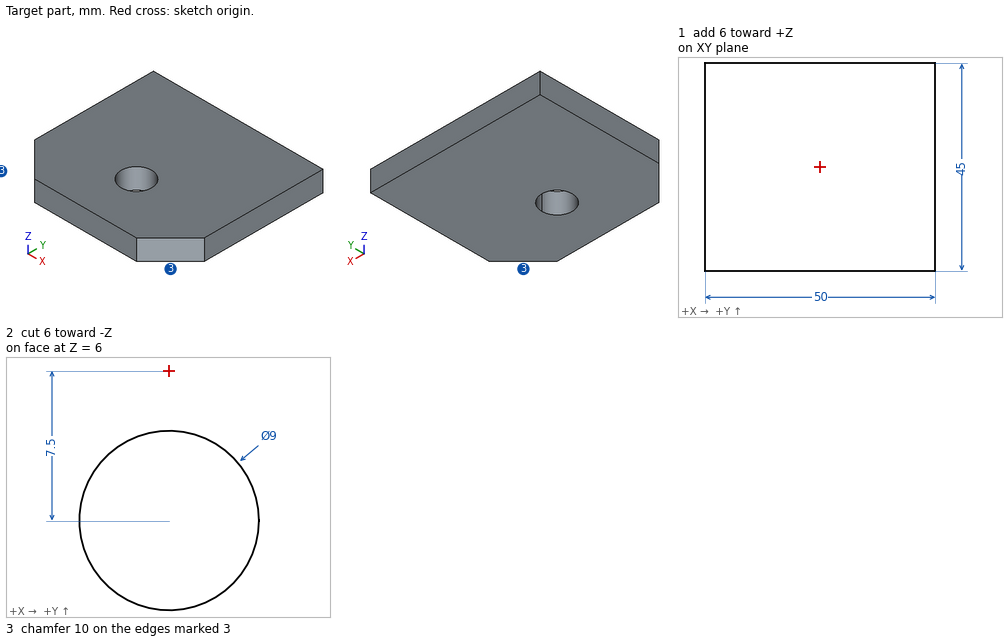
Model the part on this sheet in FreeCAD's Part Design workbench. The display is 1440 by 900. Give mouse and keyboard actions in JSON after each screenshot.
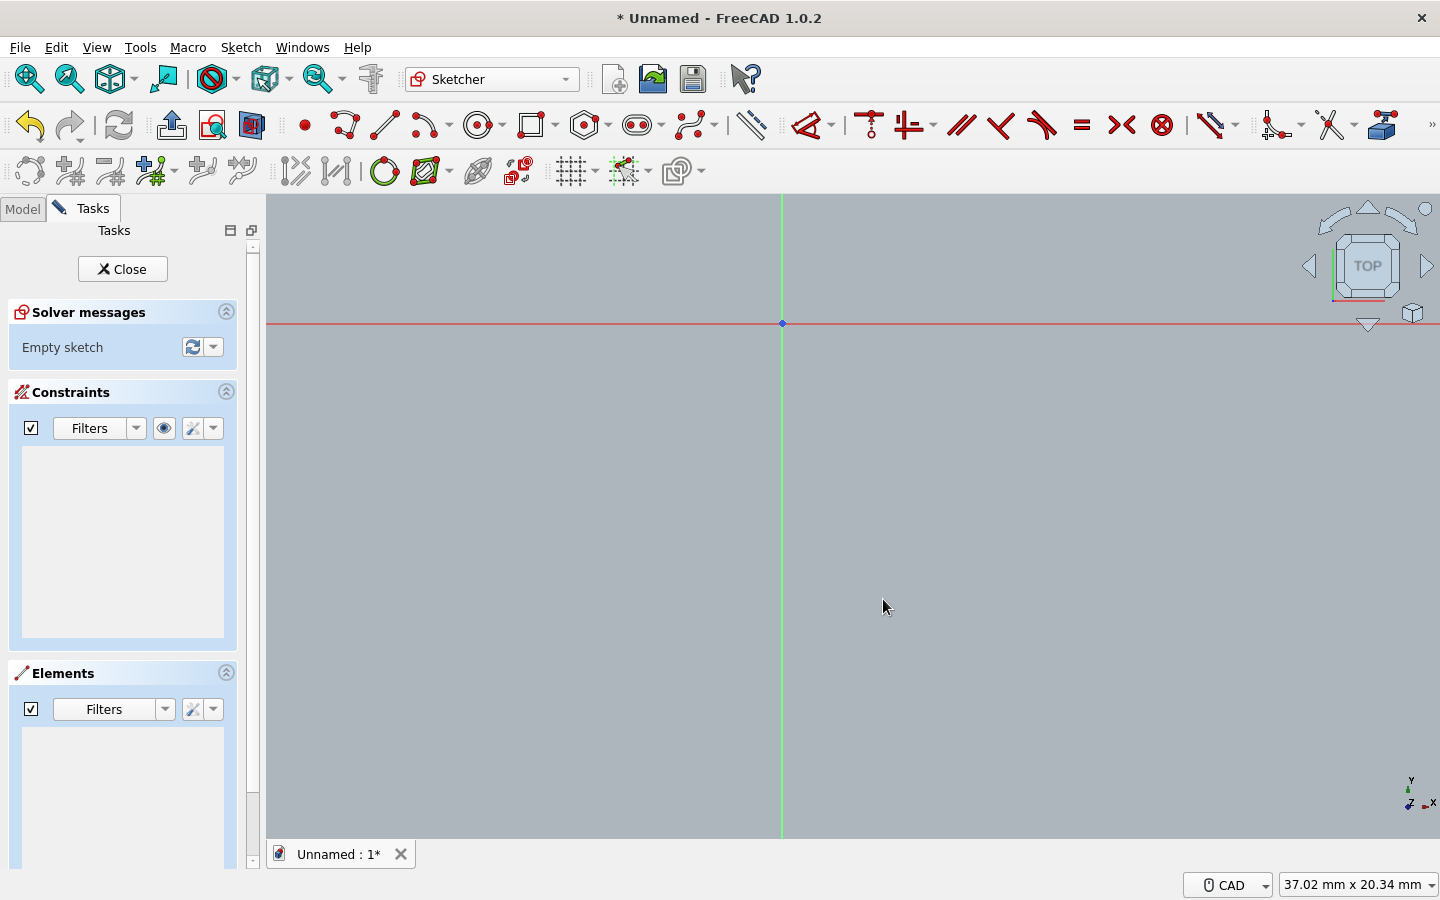
{"action": "key", "text": "g c"}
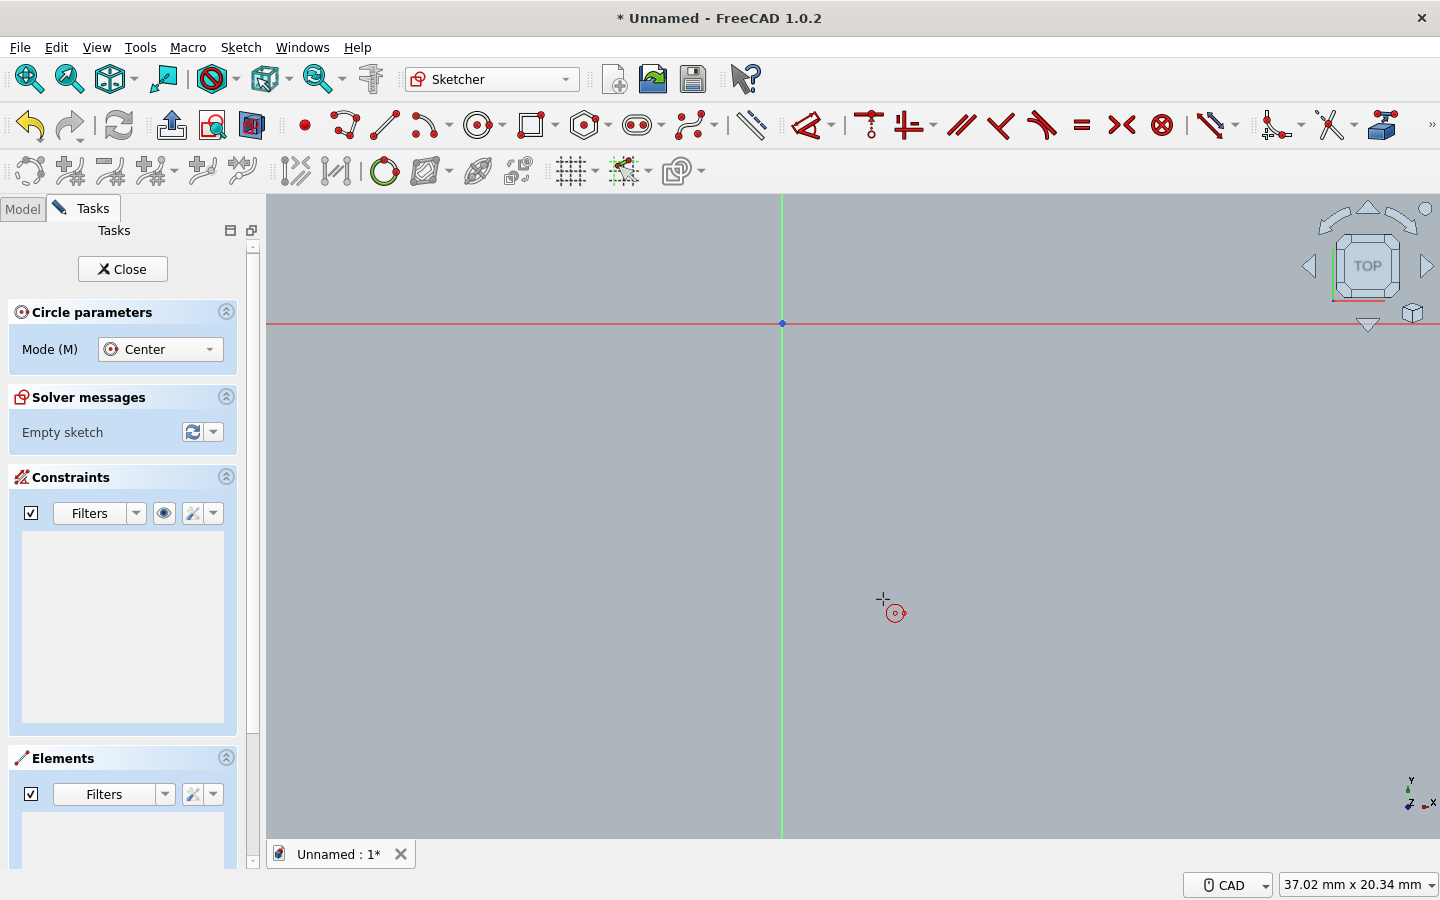
{"action": "left_click", "coordinate": [782, 561]}
{"action": "mouse_move", "coordinate": [883, 461]}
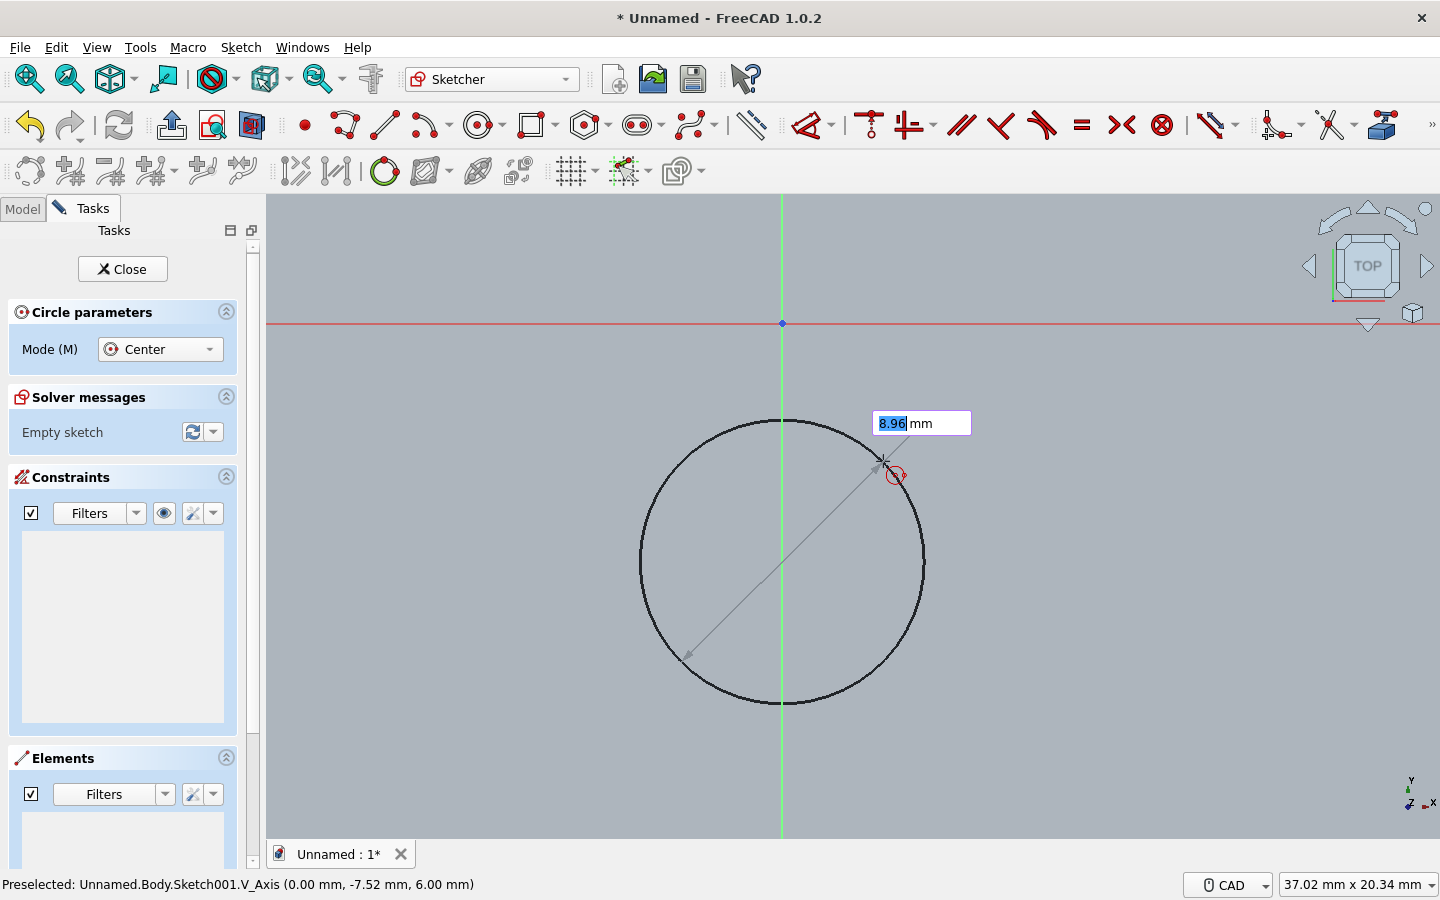
{"action": "type", "text": "9"}
{"action": "key", "text": "Return"}
{"action": "key", "text": "Escape"}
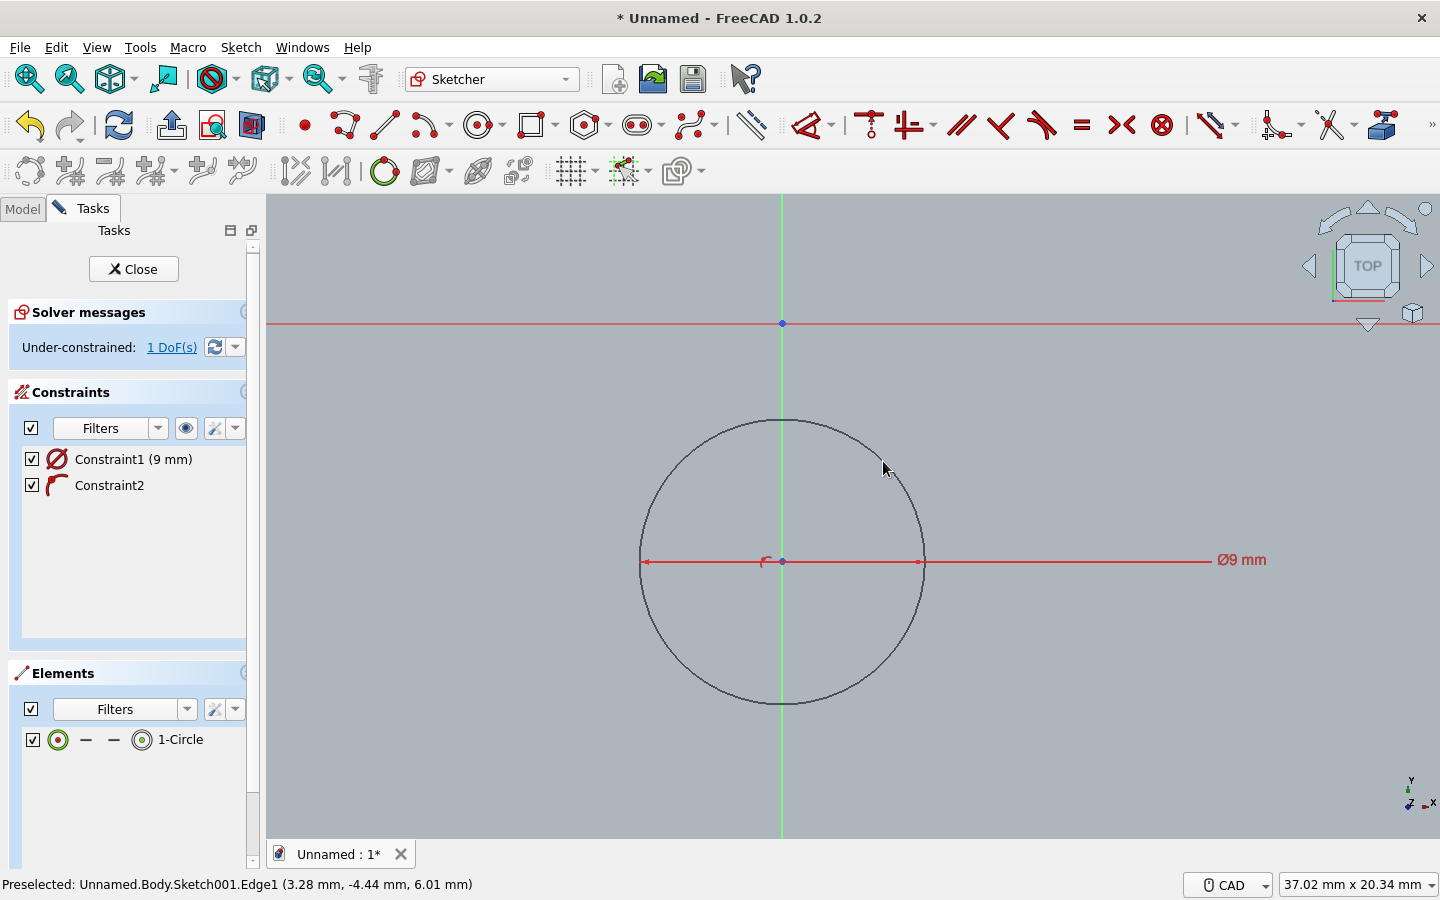
{"action": "left_click", "coordinate": [806, 126]}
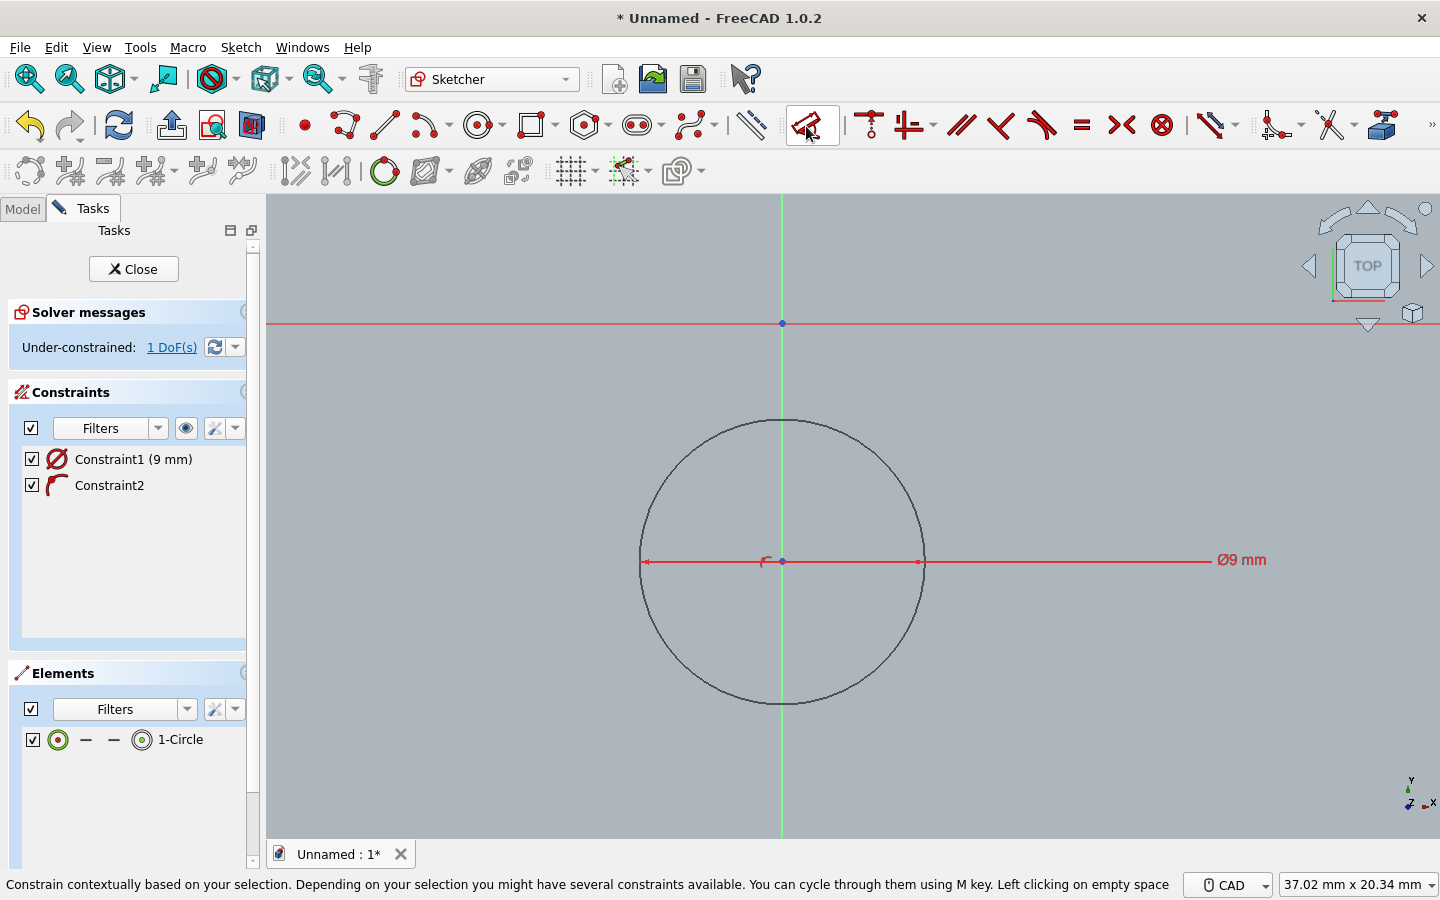
{"action": "left_click", "coordinate": [782, 562]}
{"action": "left_click", "coordinate": [816, 443]}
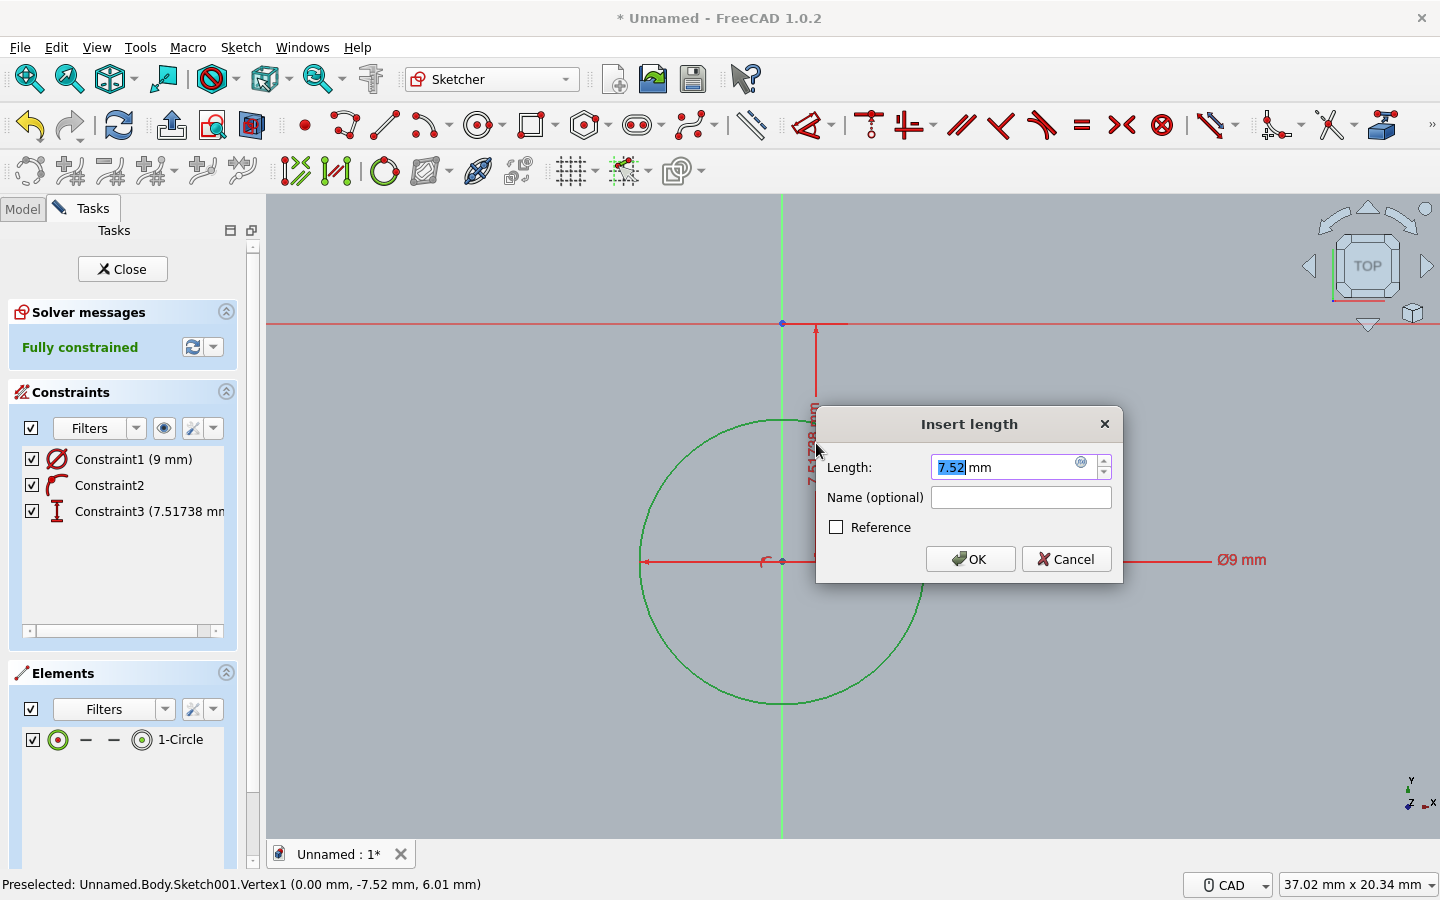
{"action": "type", "text": "7.5"}
{"action": "key", "text": "Return"}
{"action": "key", "text": "Escape"}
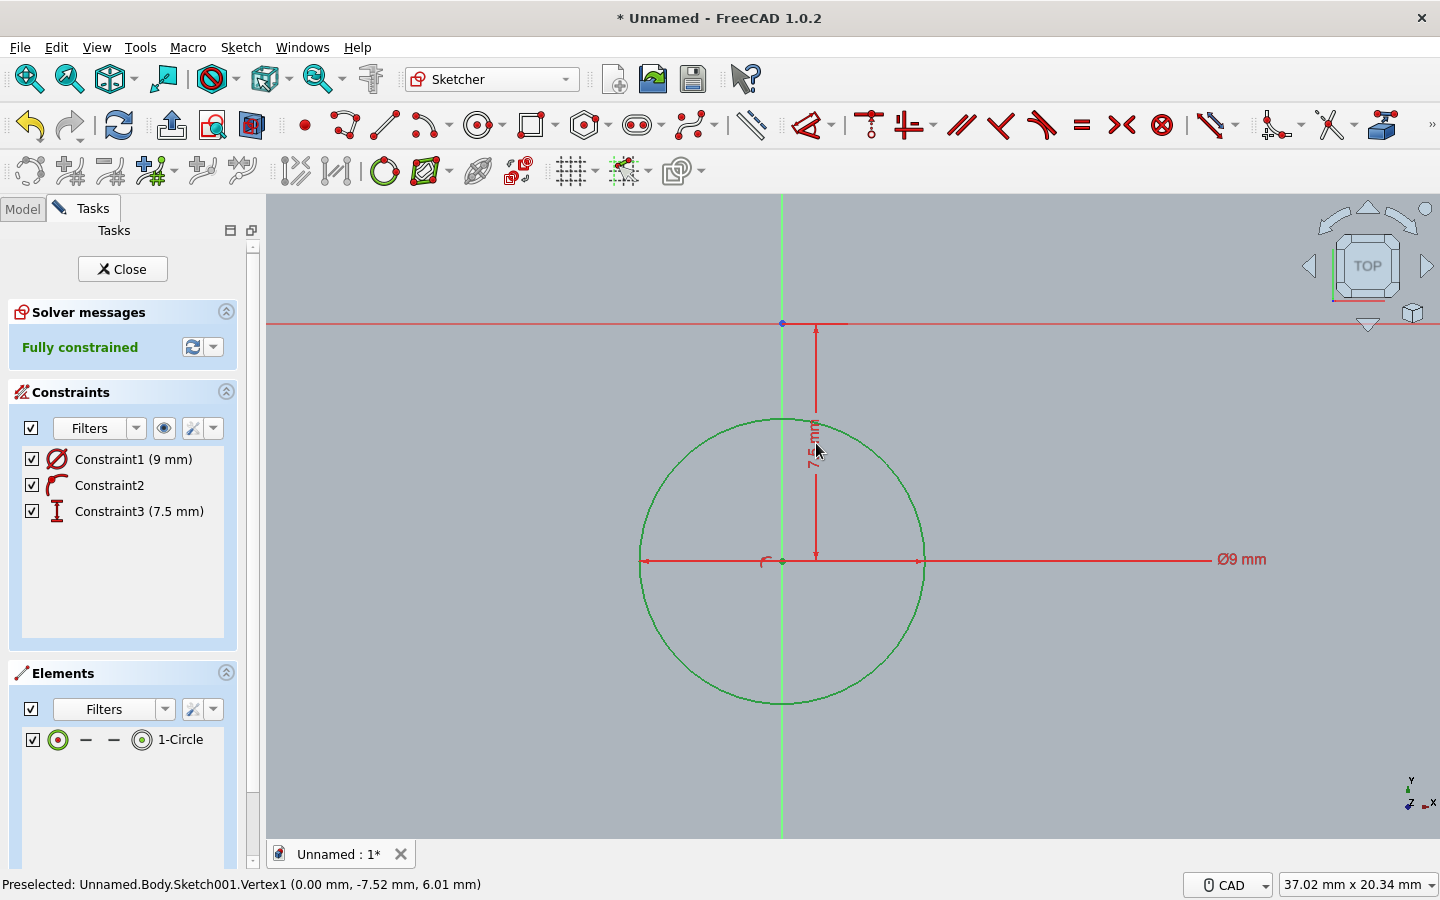
{"action": "left_click", "coordinate": [123, 269]}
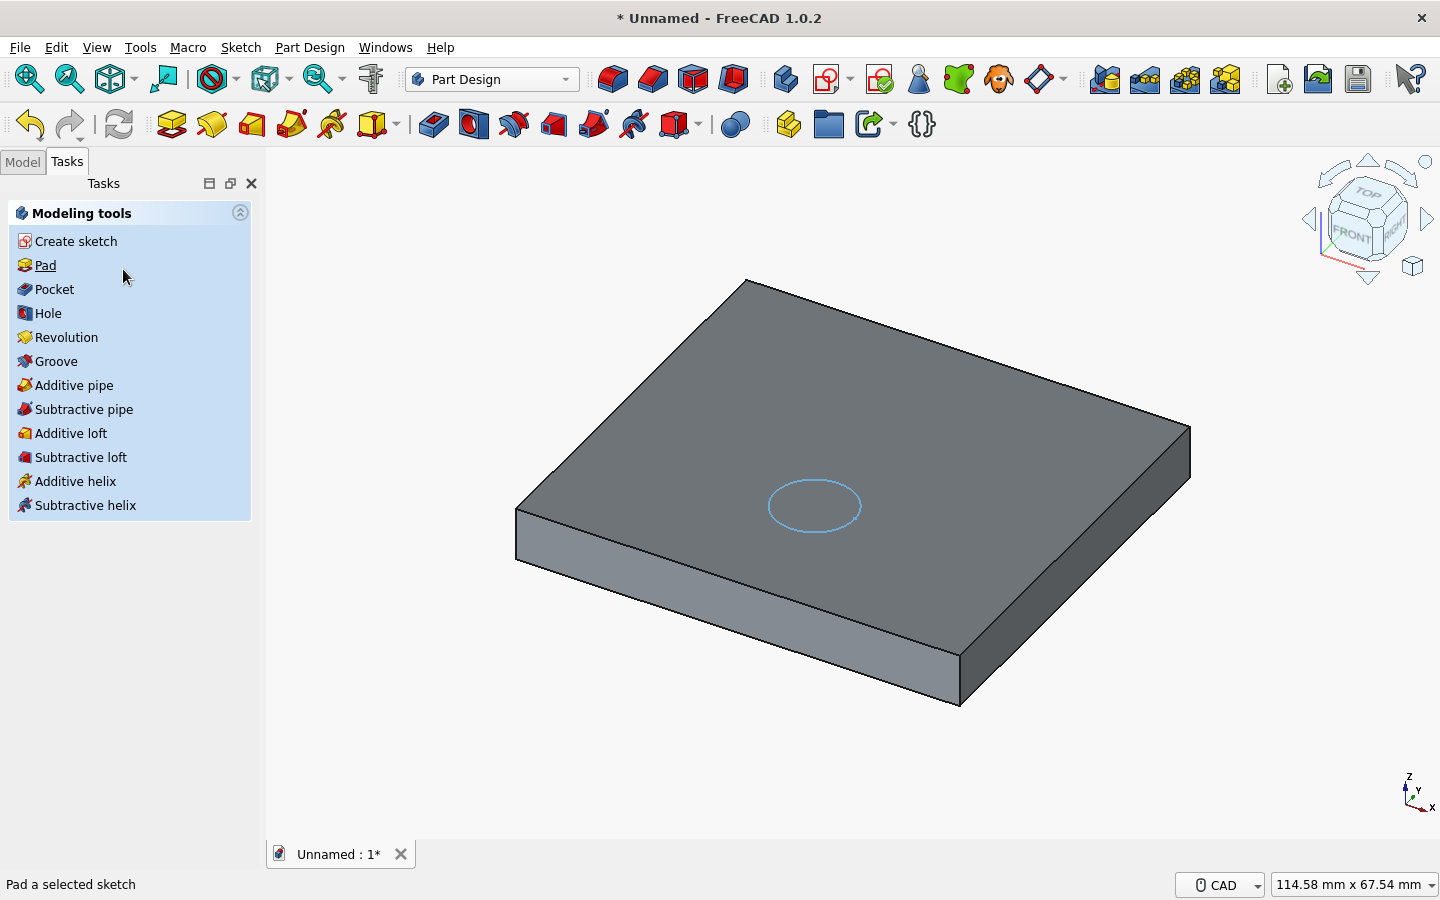
{"action": "left_click", "coordinate": [434, 124]}